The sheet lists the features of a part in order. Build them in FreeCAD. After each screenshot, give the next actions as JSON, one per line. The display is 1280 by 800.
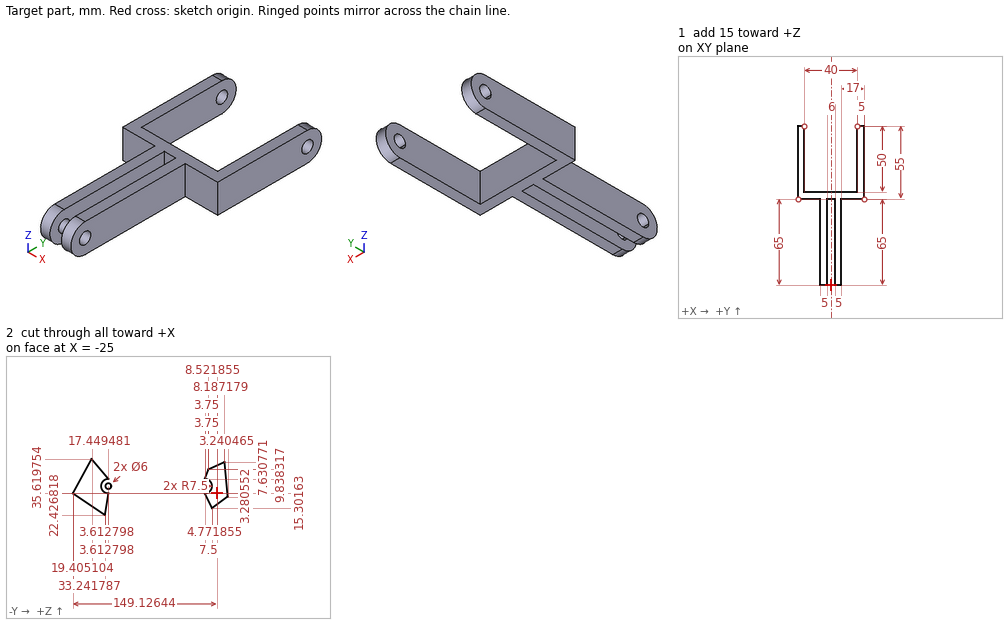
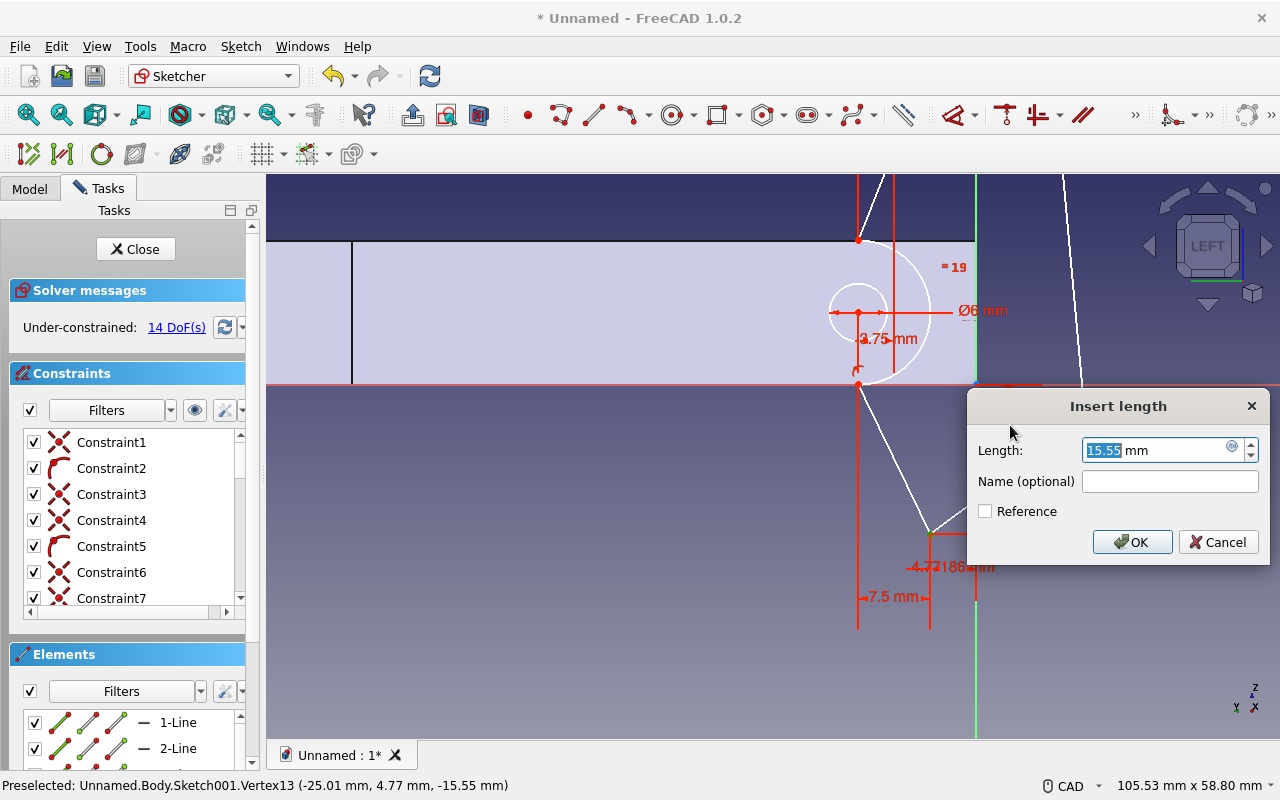
{"action": "type", "text": "15.30163"}
{"action": "key", "text": "Return"}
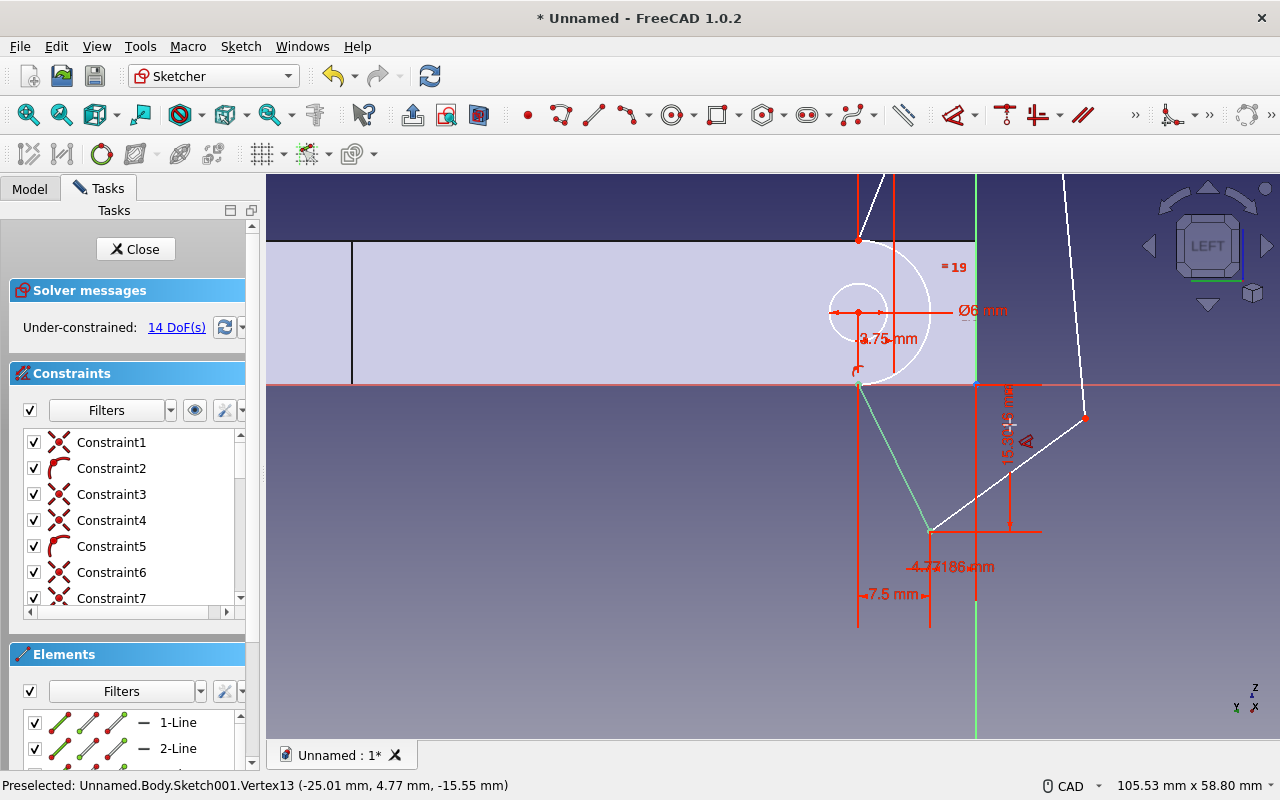
{"action": "scroll", "coordinate": [1085, 418], "scroll_direction": "up", "scroll_amount": 2}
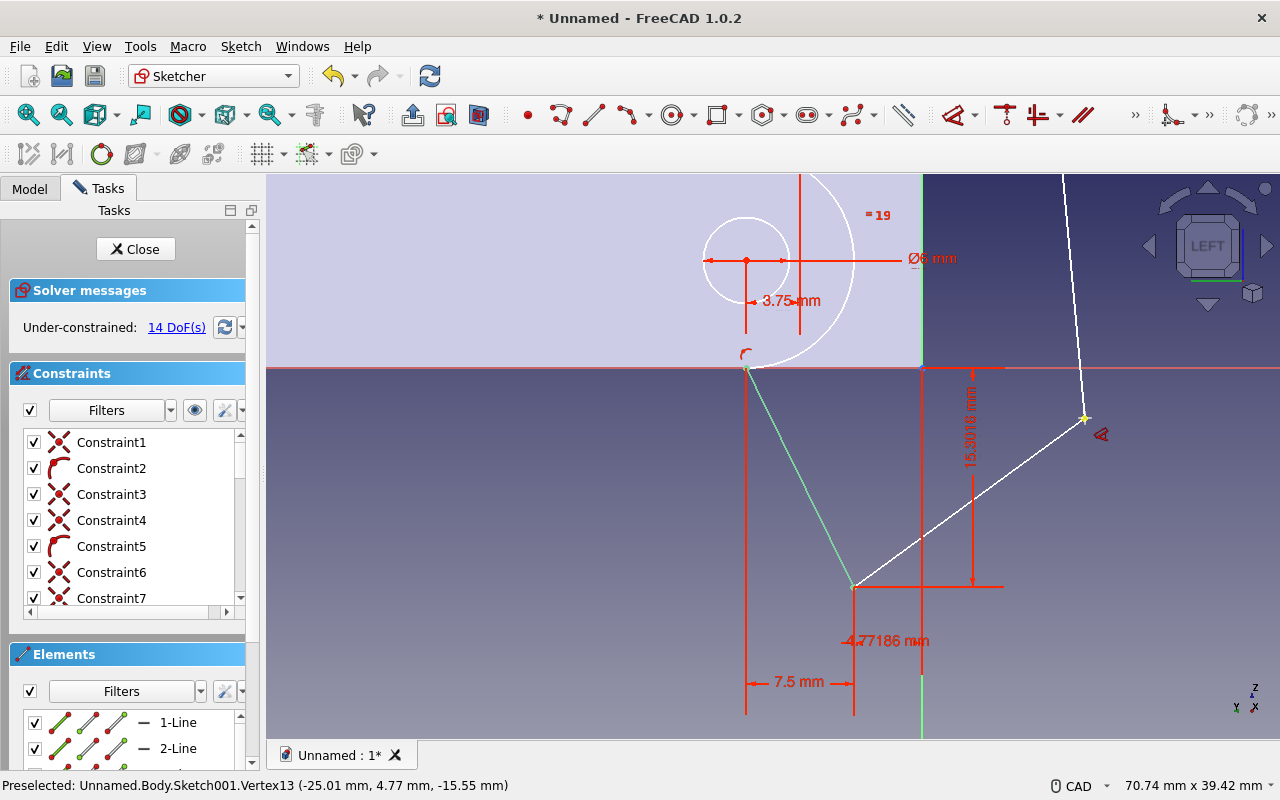
{"action": "left_click", "coordinate": [1085, 418]}
{"action": "left_click", "coordinate": [888, 393]}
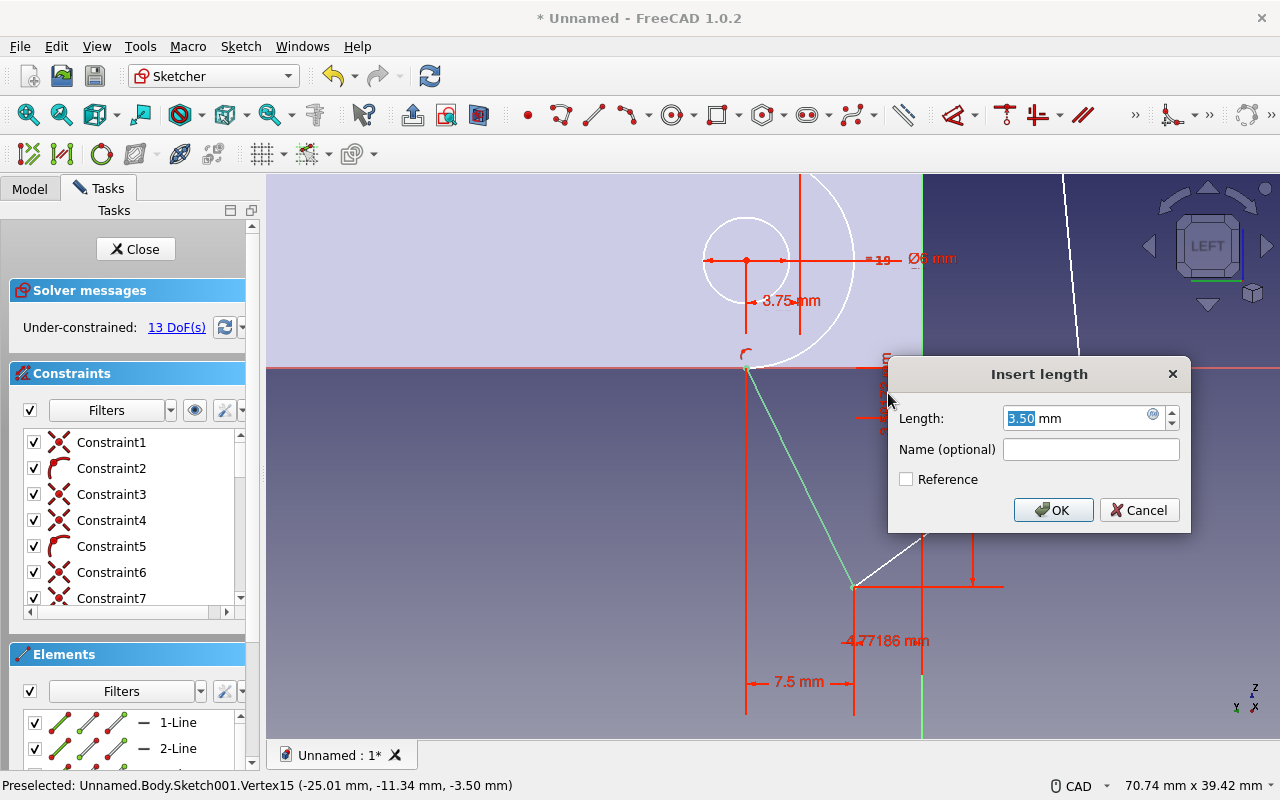
{"action": "type", "text": "3.280552"}
{"action": "key", "text": "Return"}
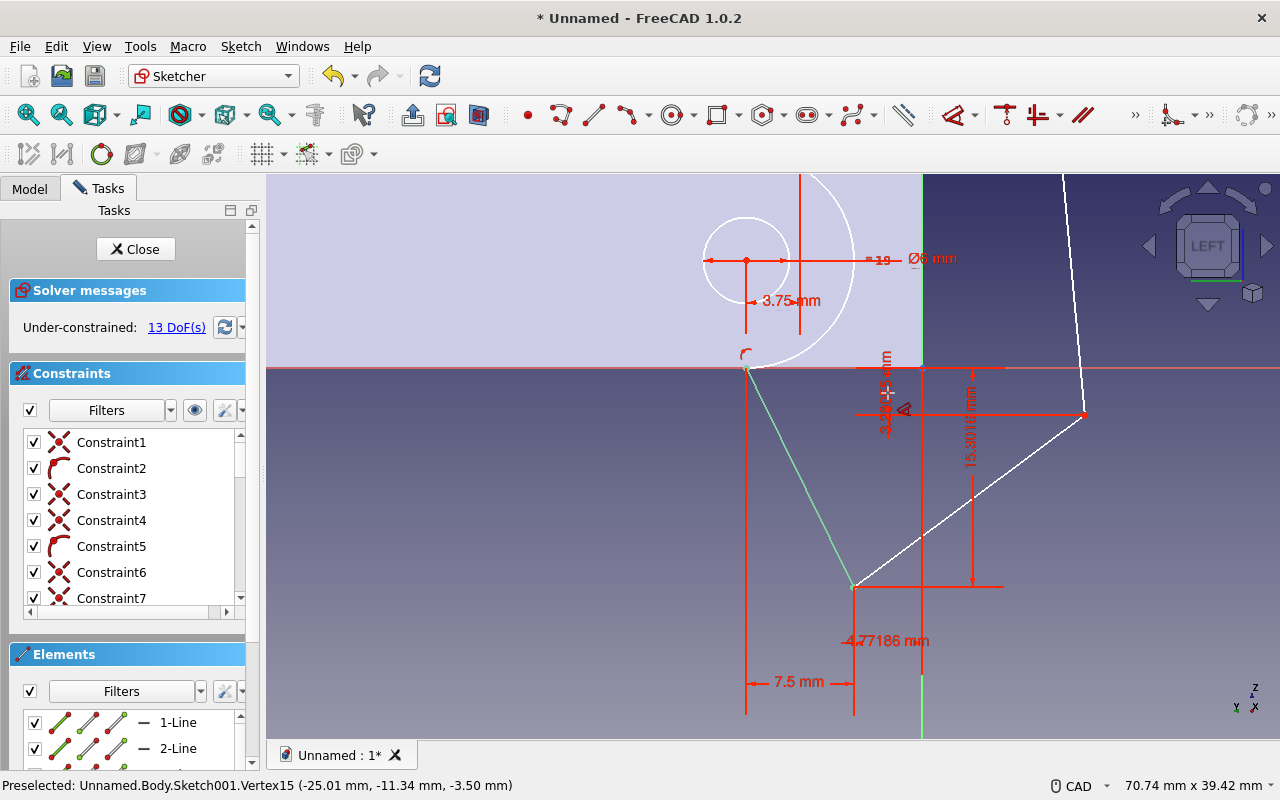
{"action": "scroll", "coordinate": [956, 516], "scroll_direction": "down", "scroll_amount": 7}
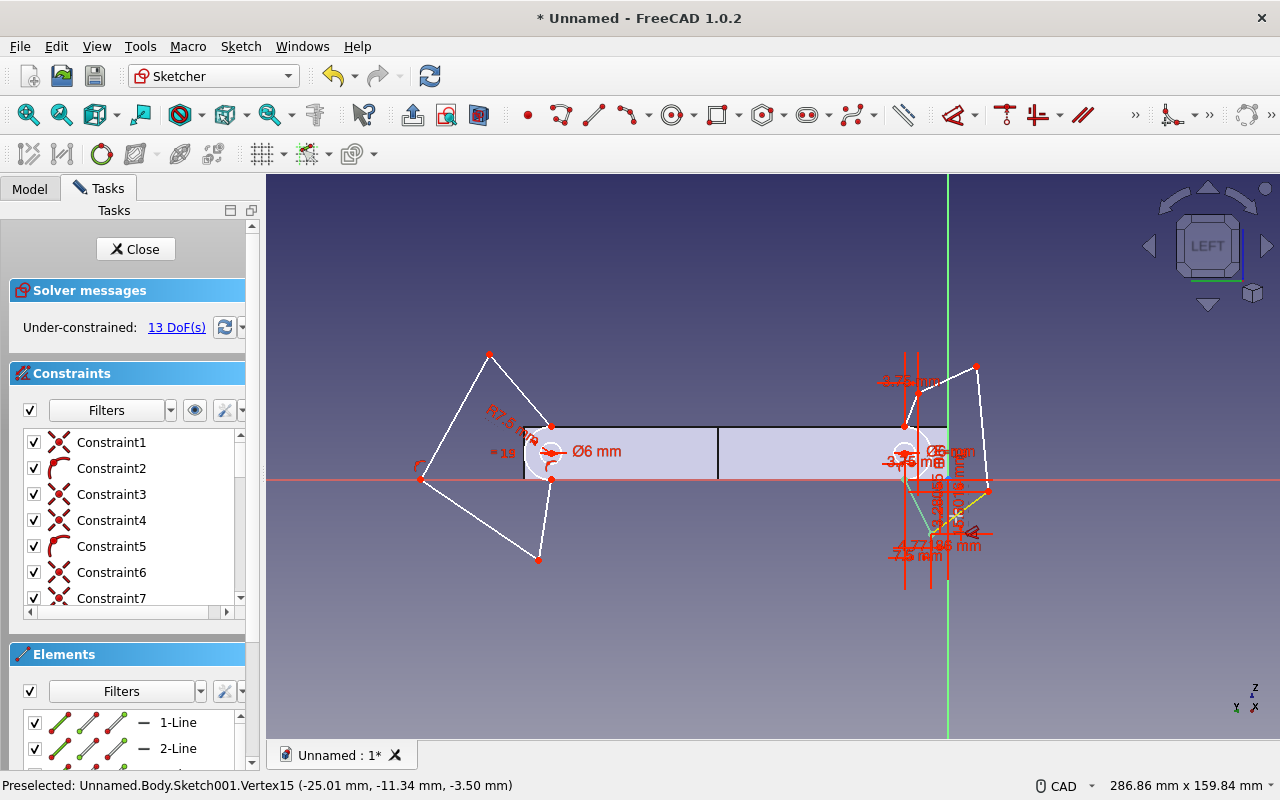
{"action": "scroll", "coordinate": [977, 366], "scroll_direction": "up", "scroll_amount": 2}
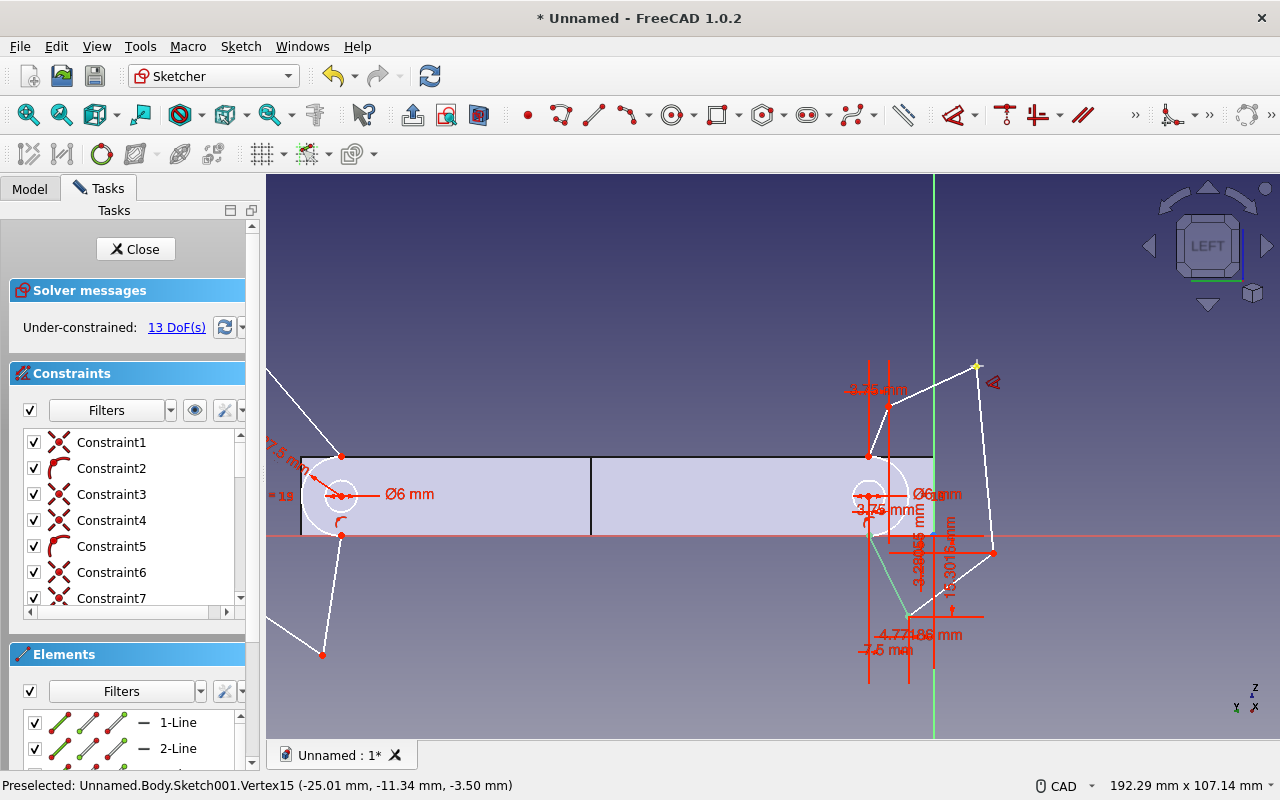
{"action": "left_click", "coordinate": [976, 366]}
{"action": "left_click", "coordinate": [955, 332]}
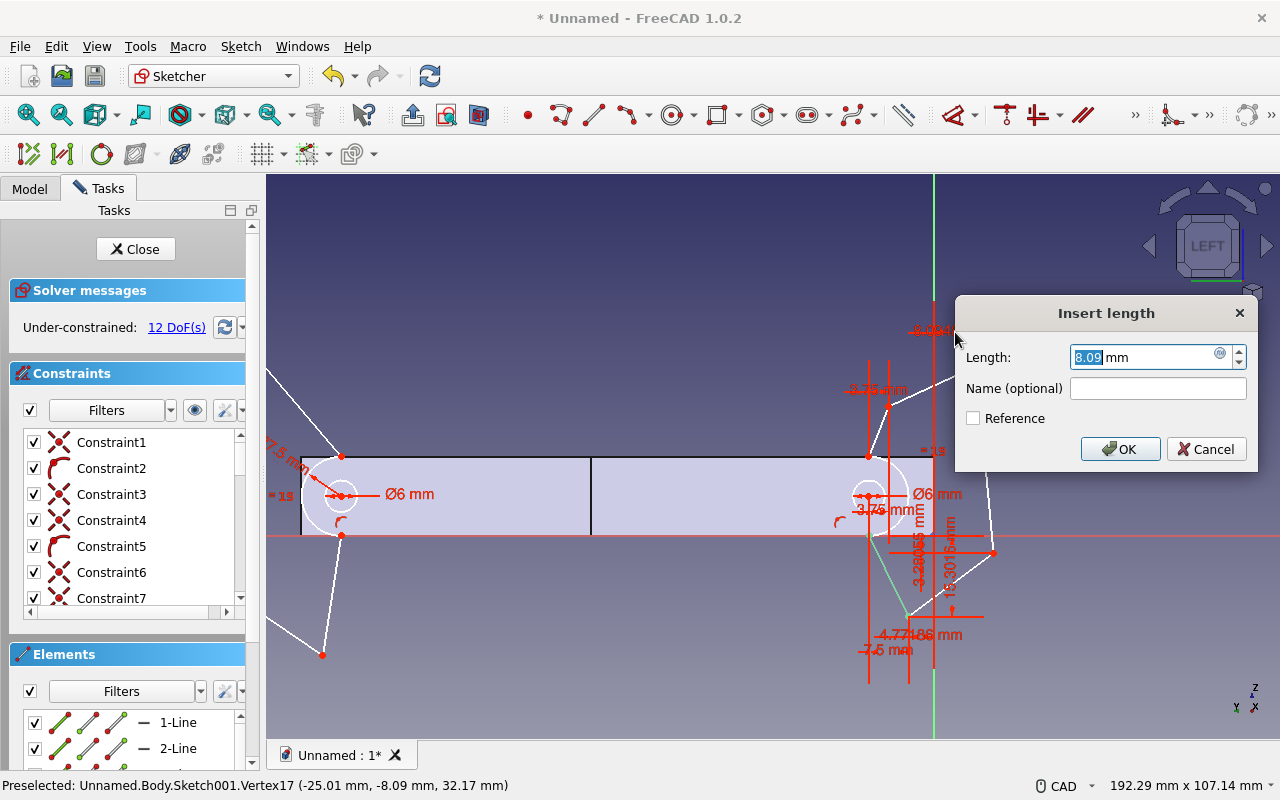
{"action": "type", "text": "8.187179"}
{"action": "key", "text": "Return"}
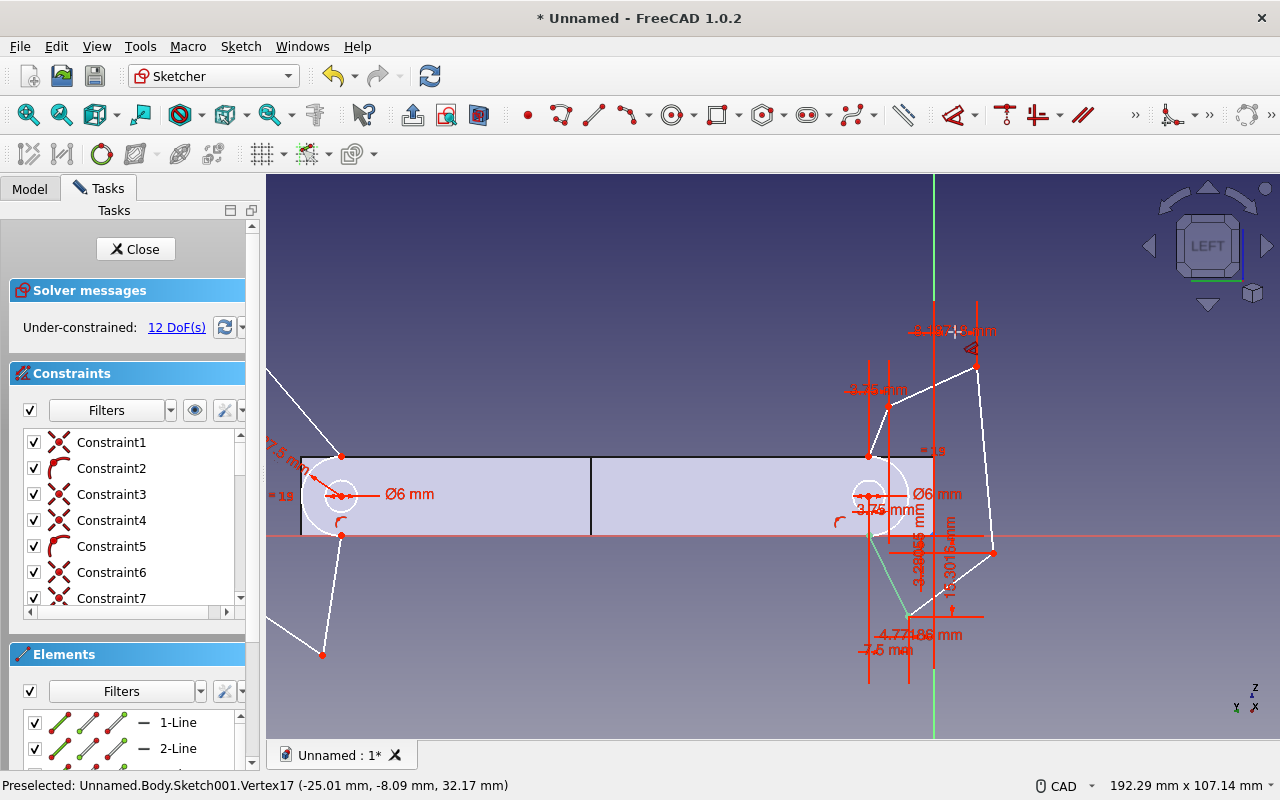
{"action": "left_click", "coordinate": [889, 407]}
{"action": "left_click", "coordinate": [911, 301]}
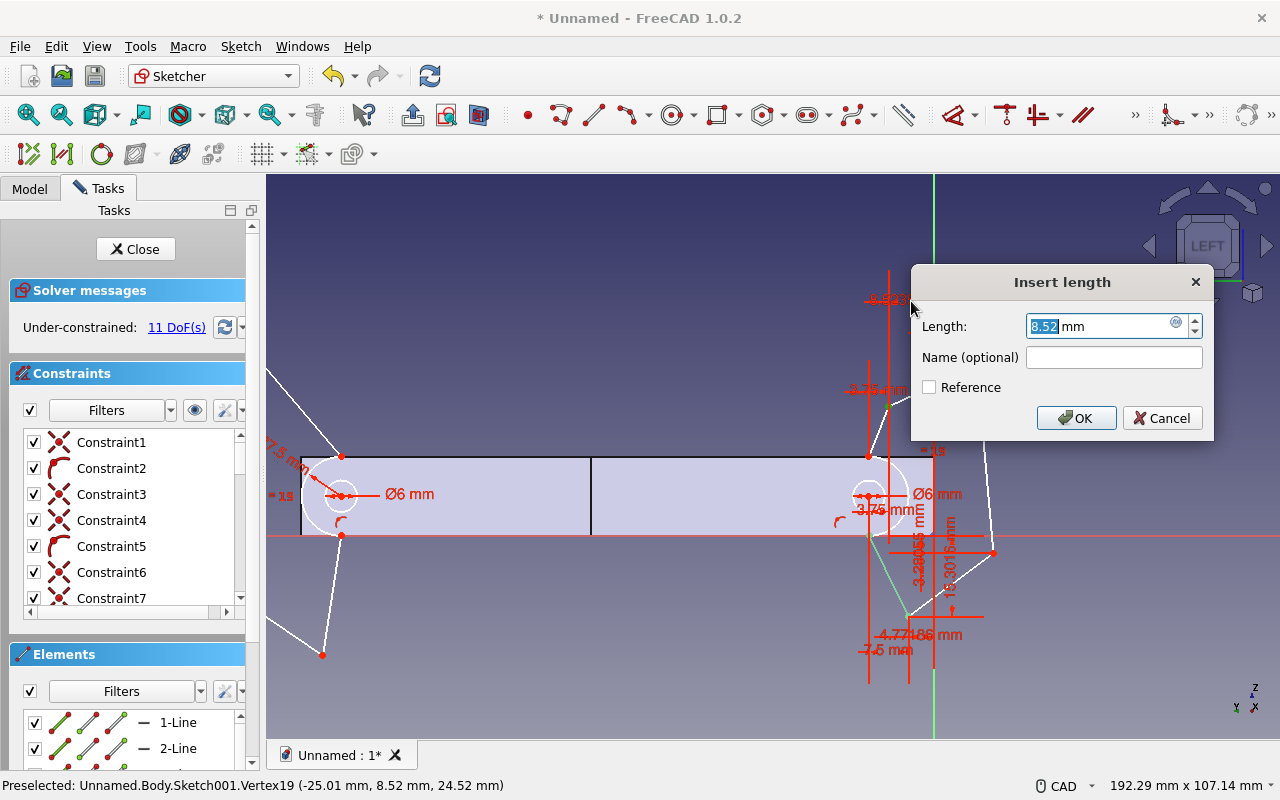
{"action": "type", "text": "8.521855"}
{"action": "key", "text": "Return"}